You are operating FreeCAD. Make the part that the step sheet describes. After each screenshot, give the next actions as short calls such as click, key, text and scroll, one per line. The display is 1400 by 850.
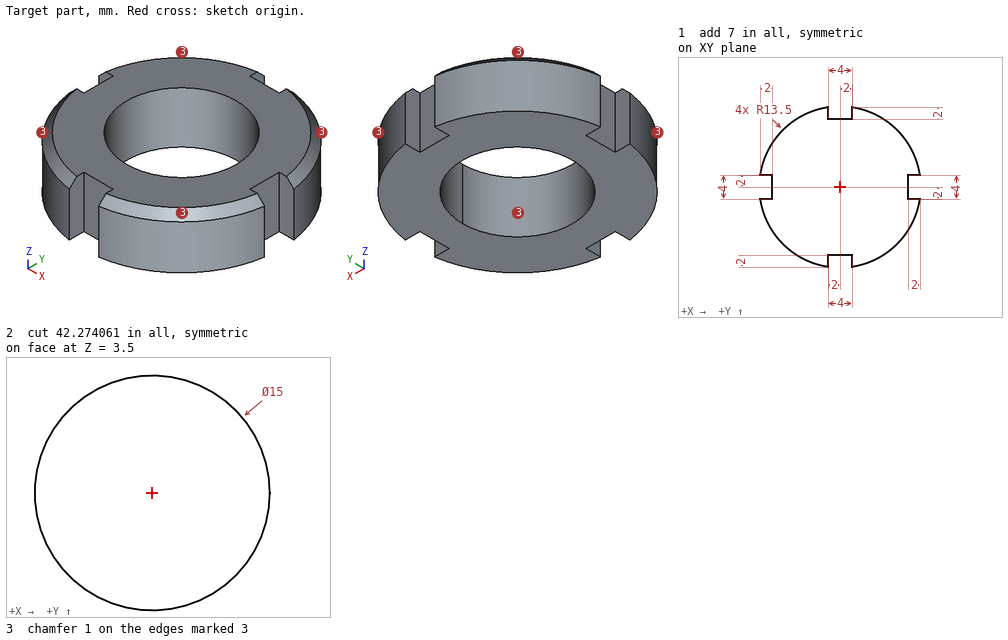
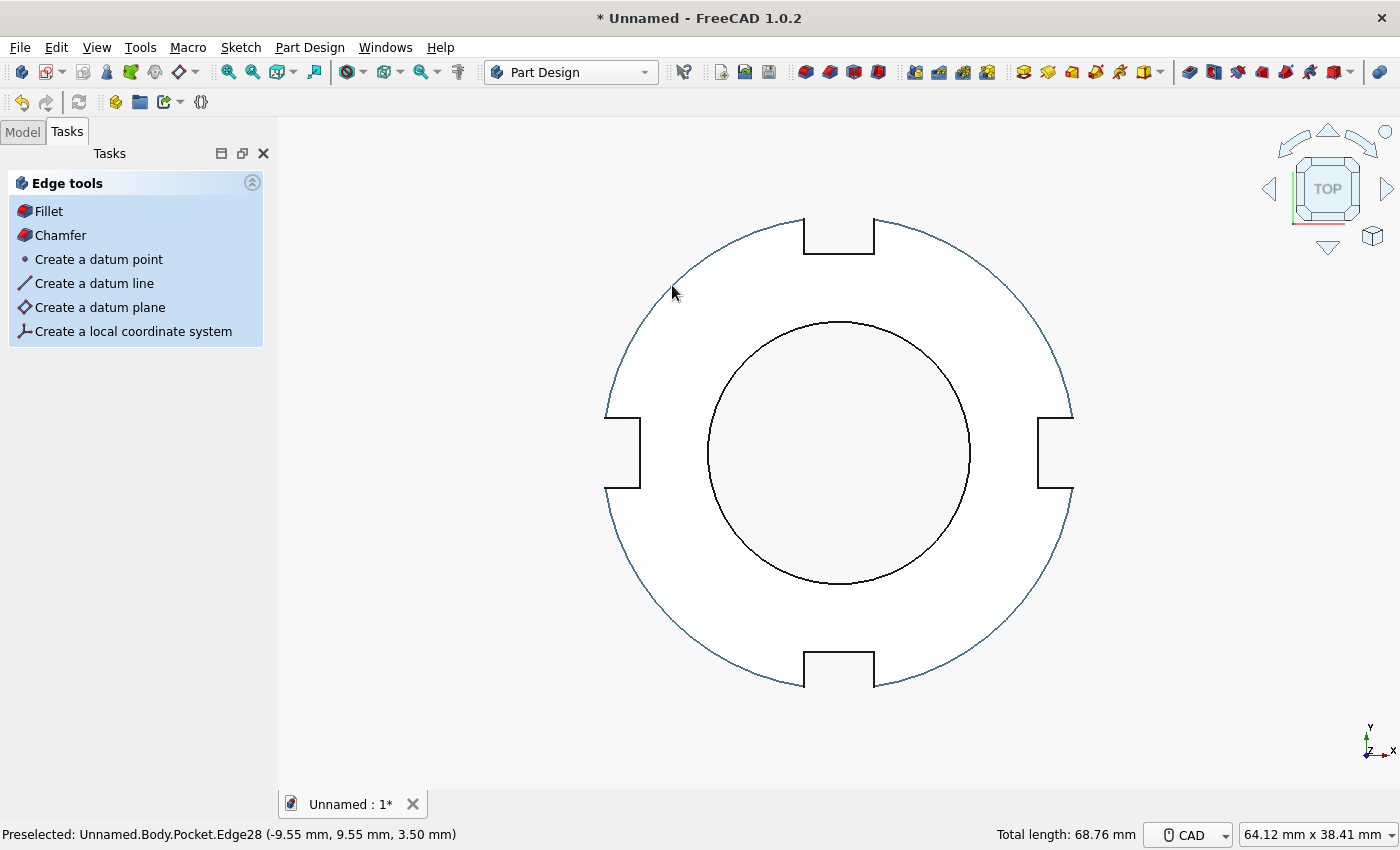
click(830, 72)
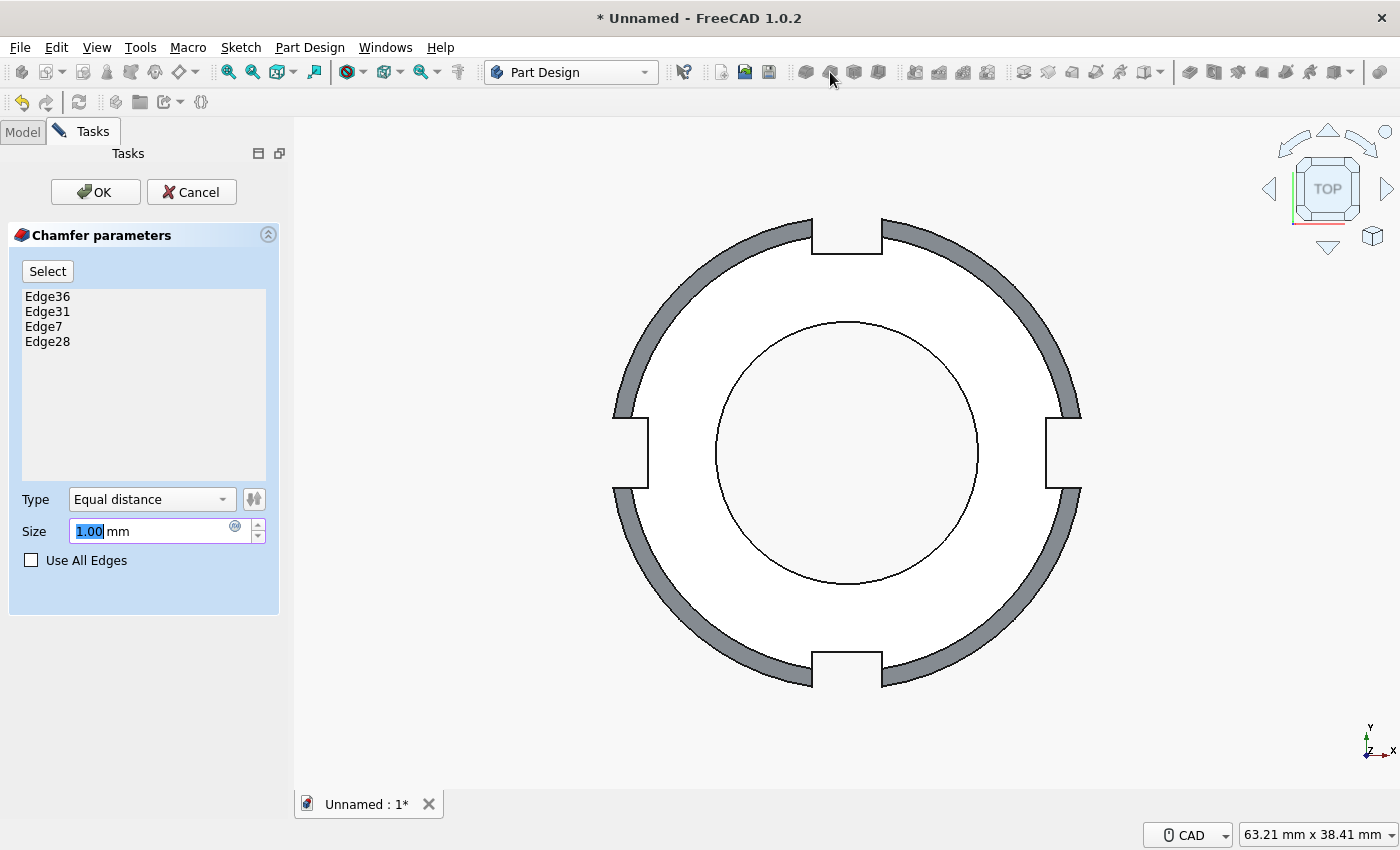
text(1)
key(Tab)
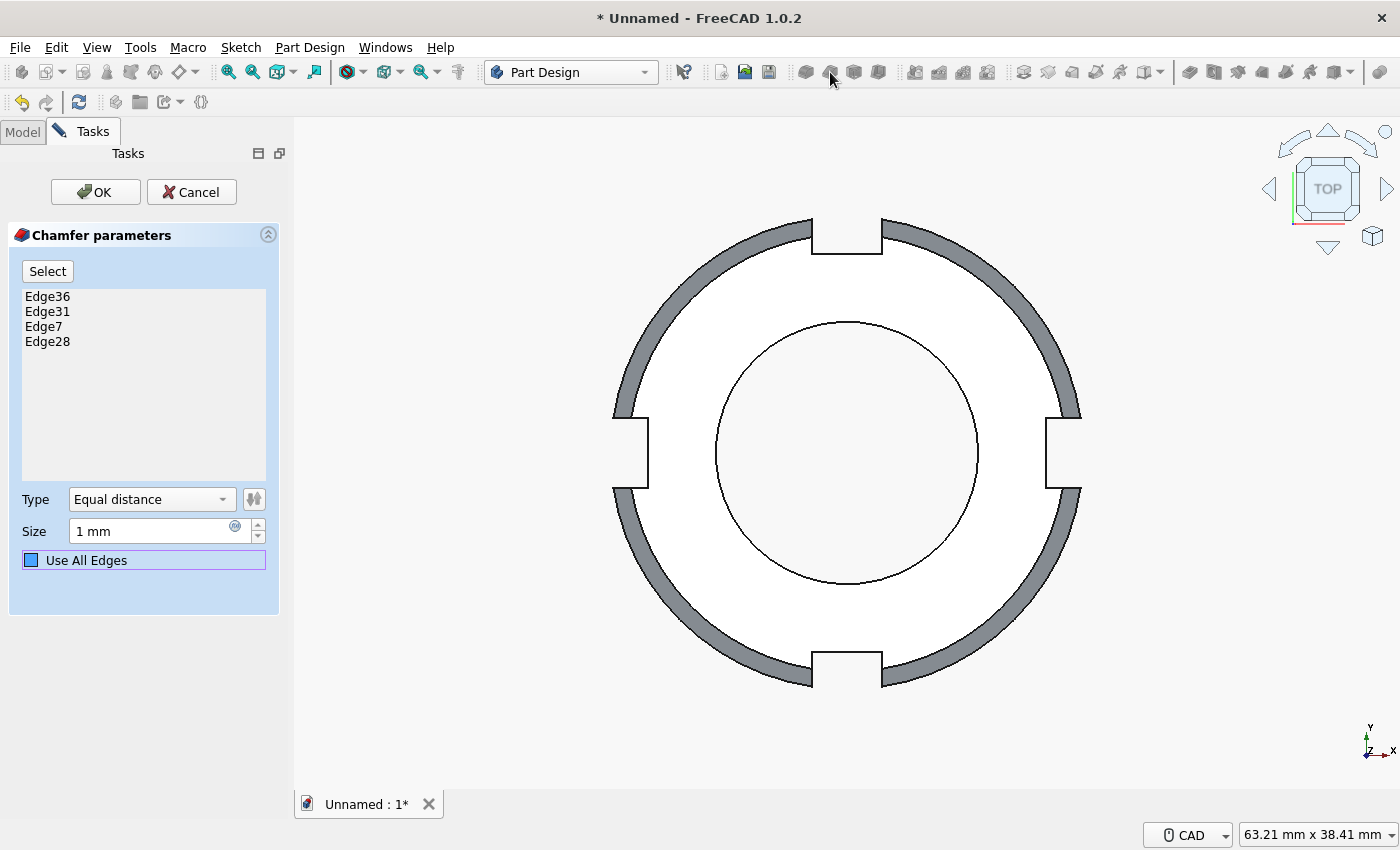
click(96, 192)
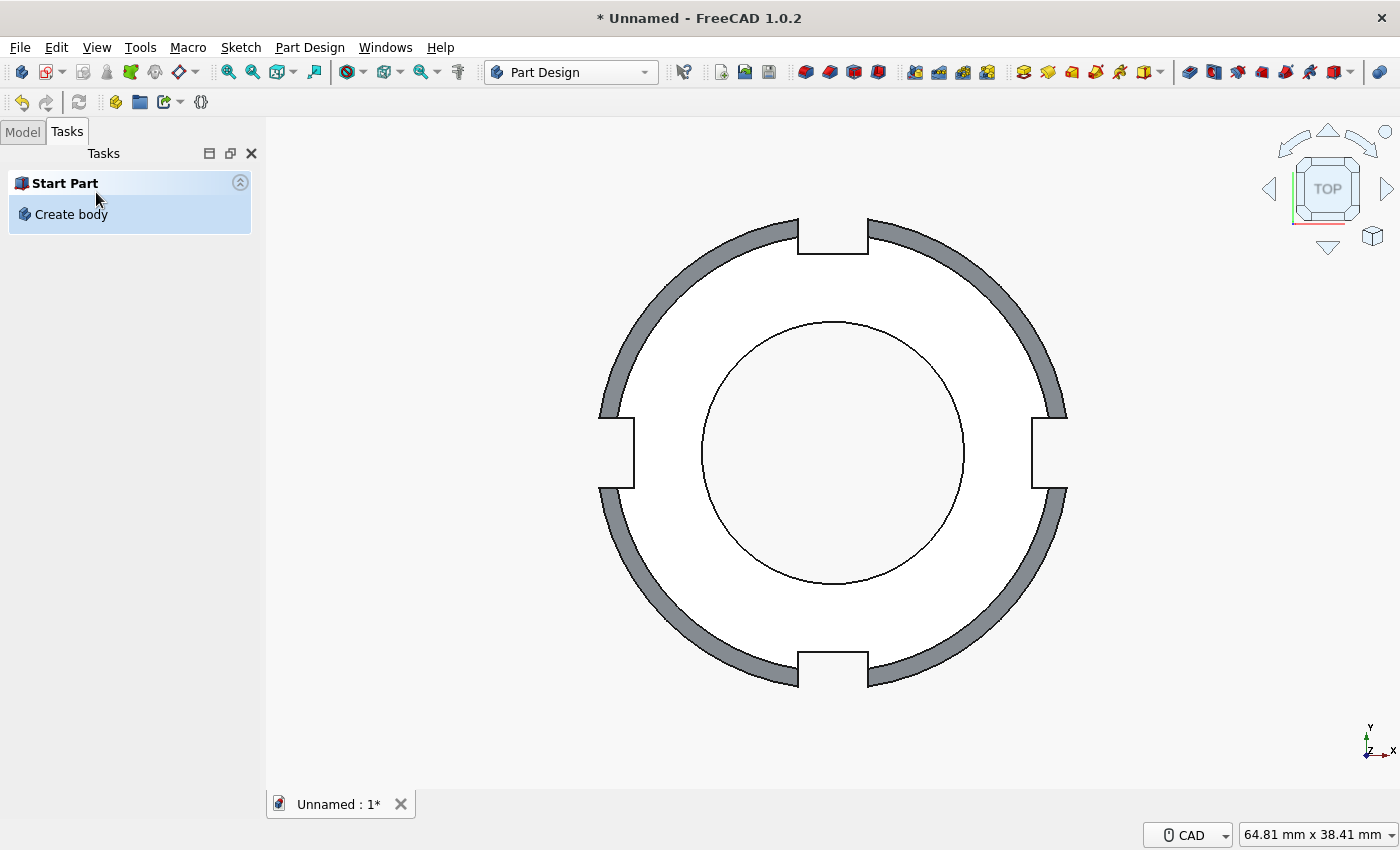
key(0)